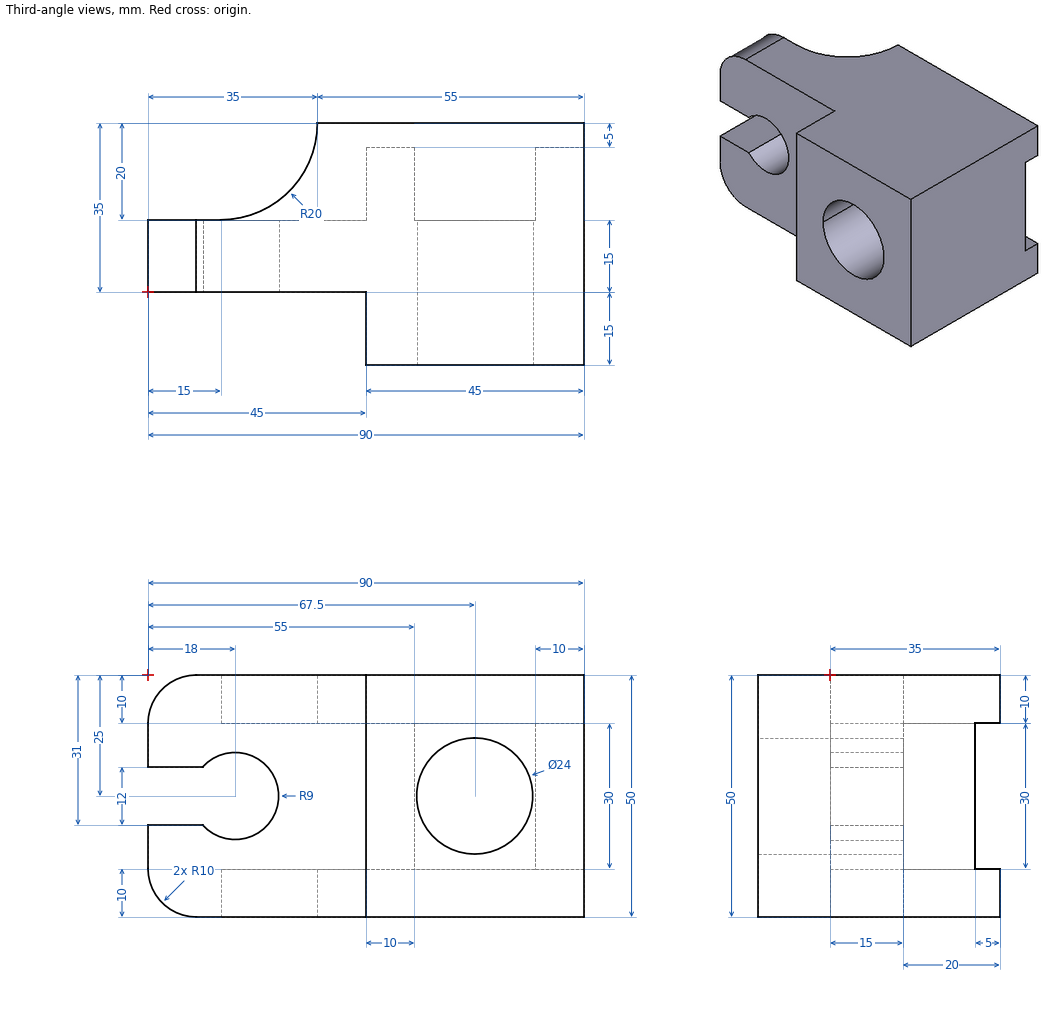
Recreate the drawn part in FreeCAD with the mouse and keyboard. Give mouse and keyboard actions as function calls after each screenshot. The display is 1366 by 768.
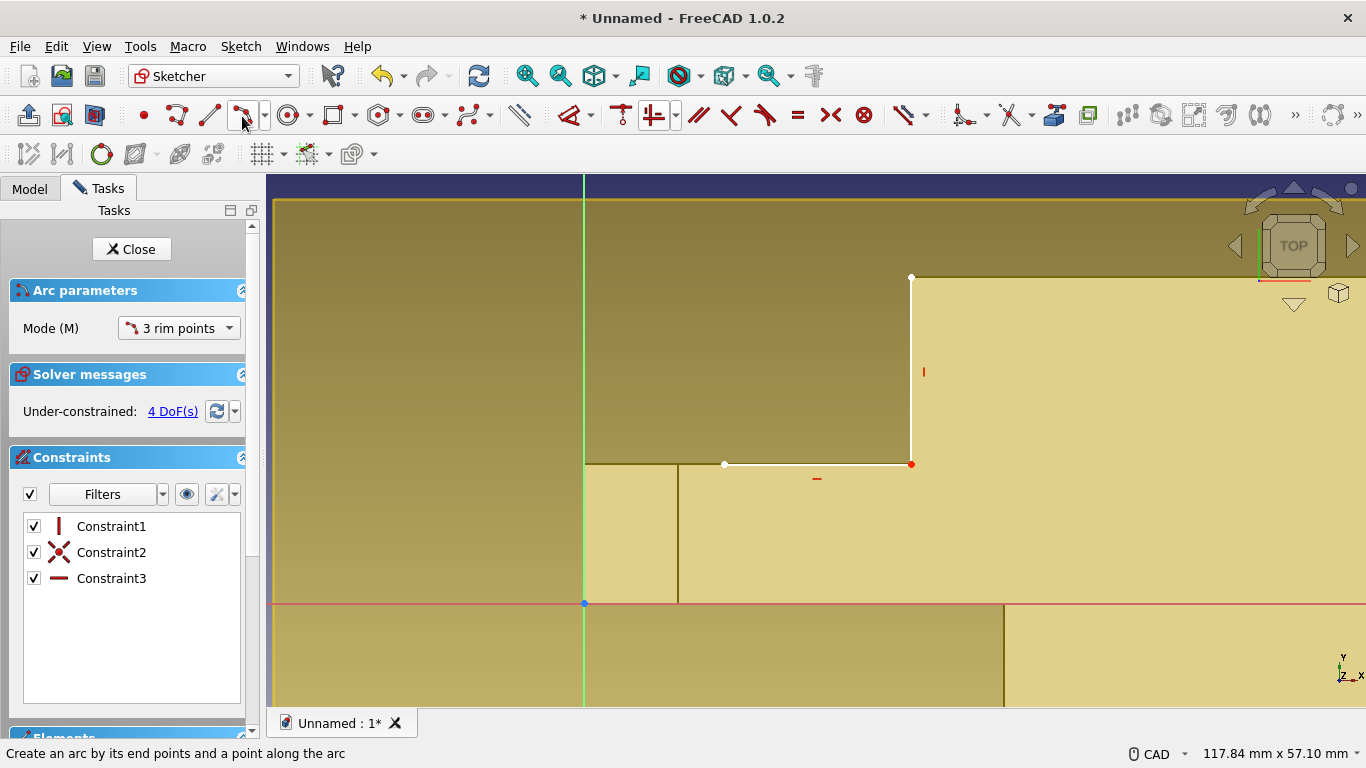
click(724, 465)
click(911, 278)
click(856, 409)
key(Escape)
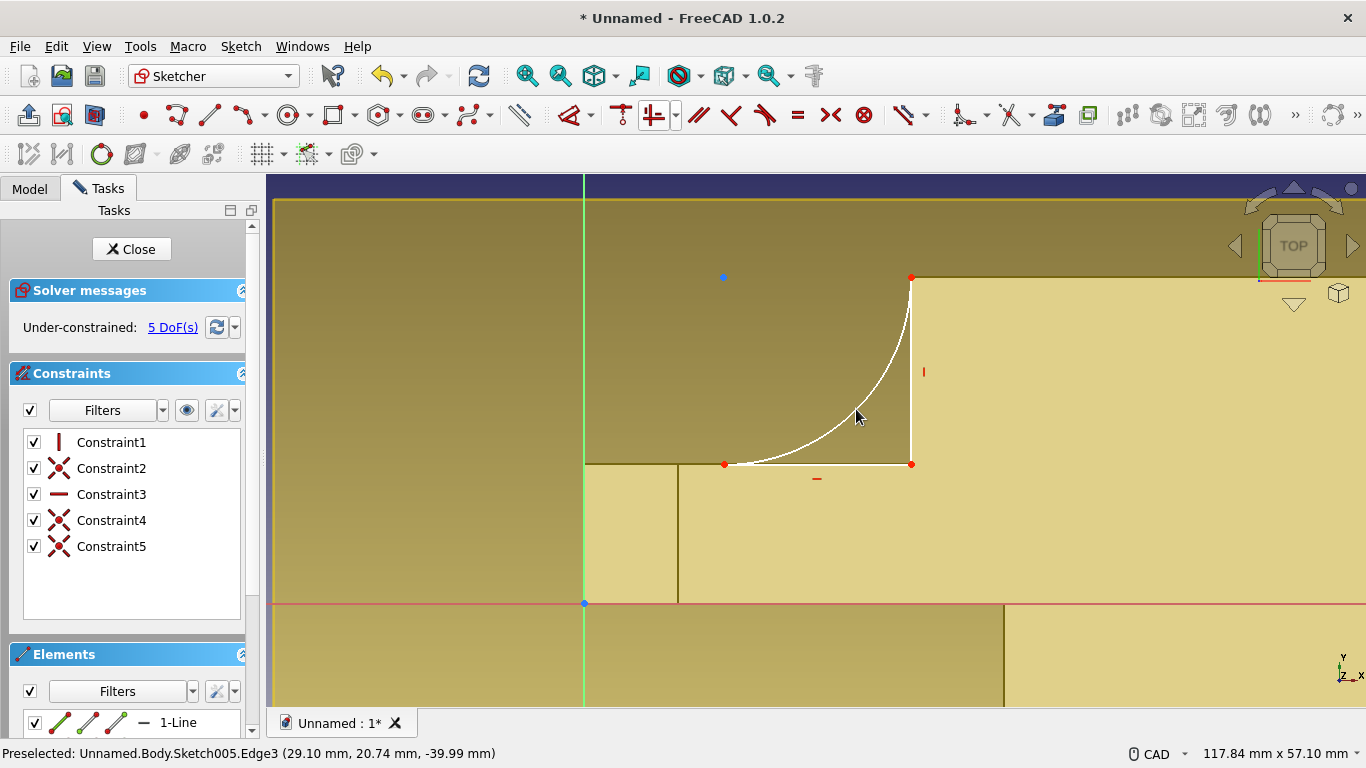
click(911, 409)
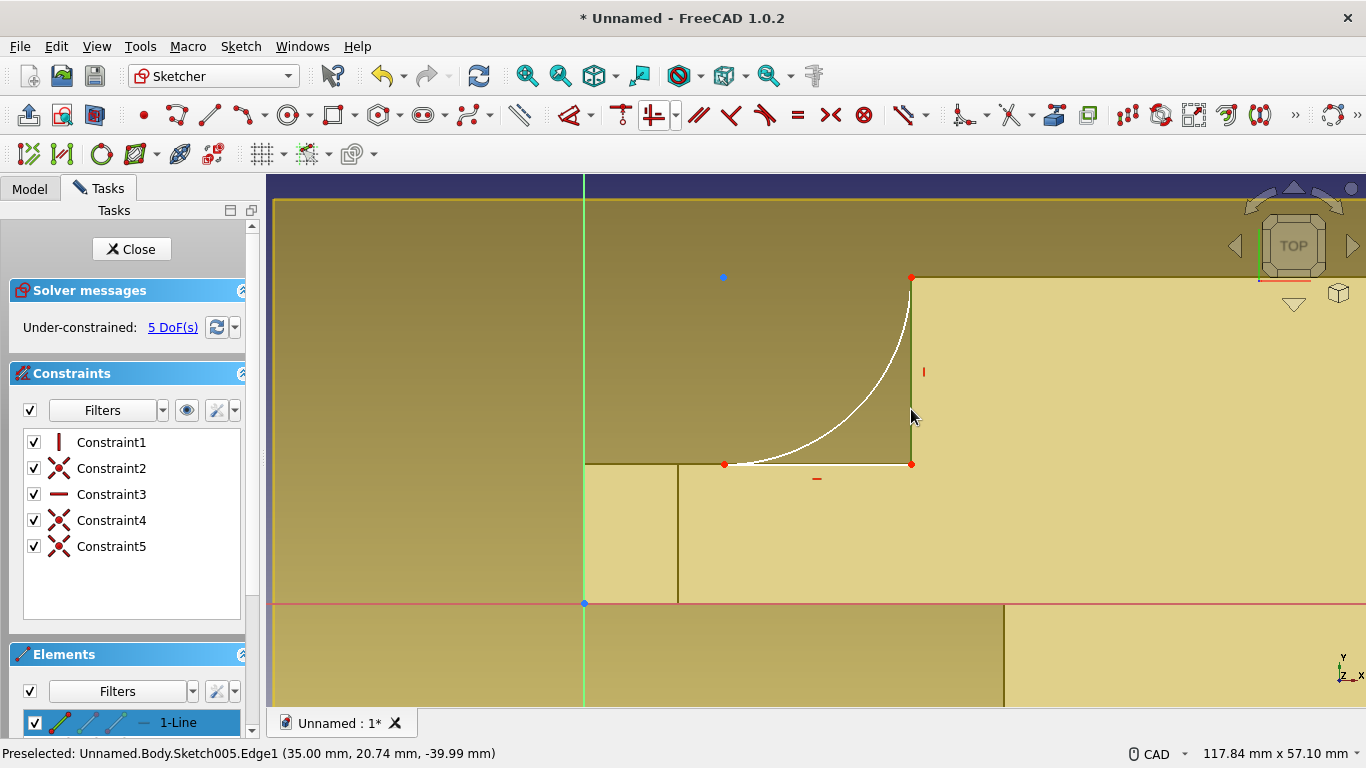
click(809, 444)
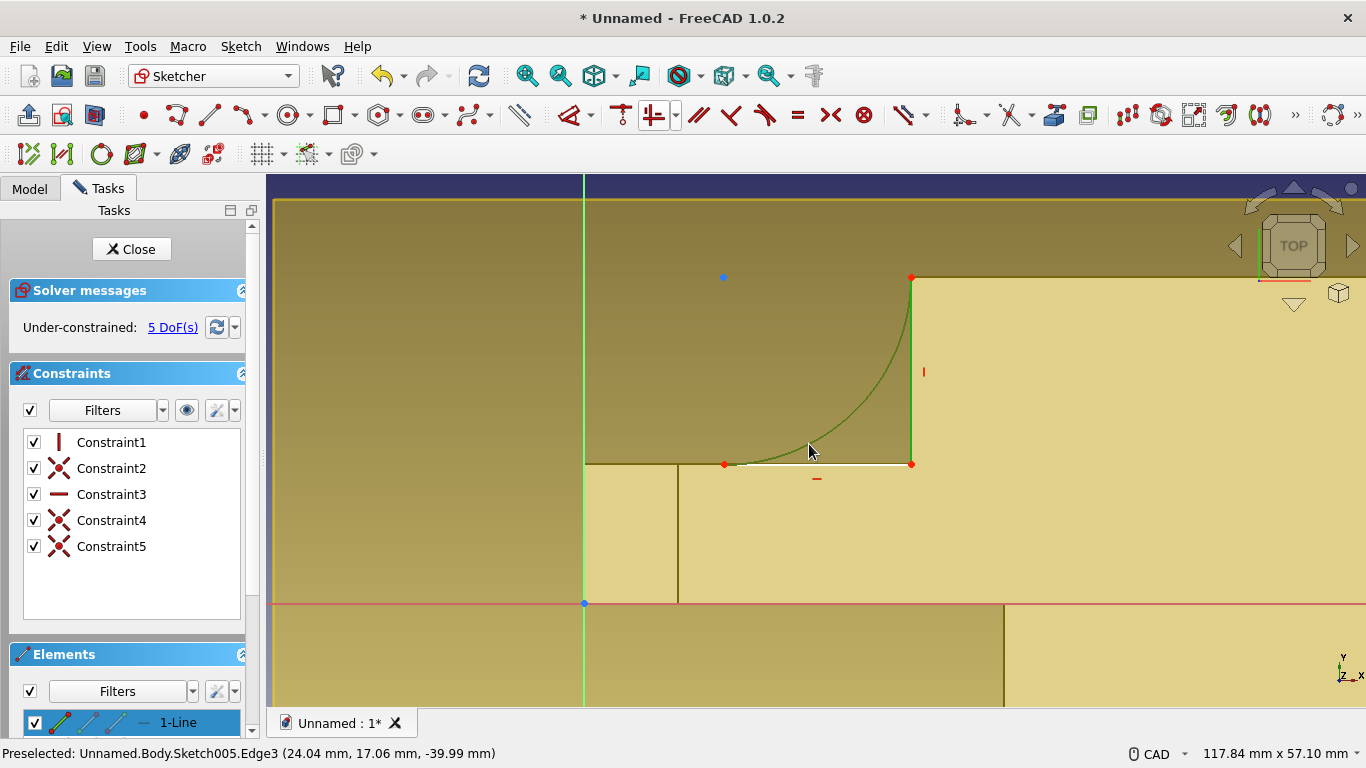
key(t)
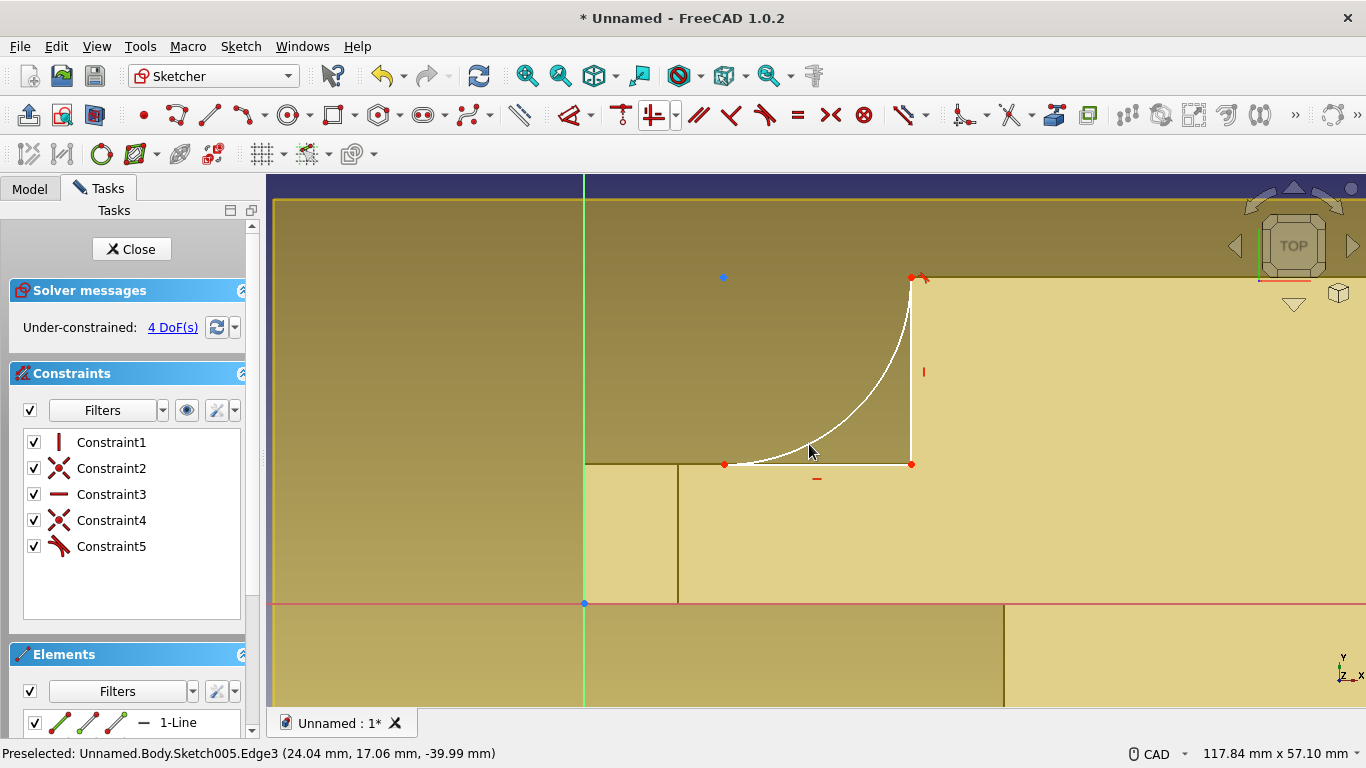
click(855, 465)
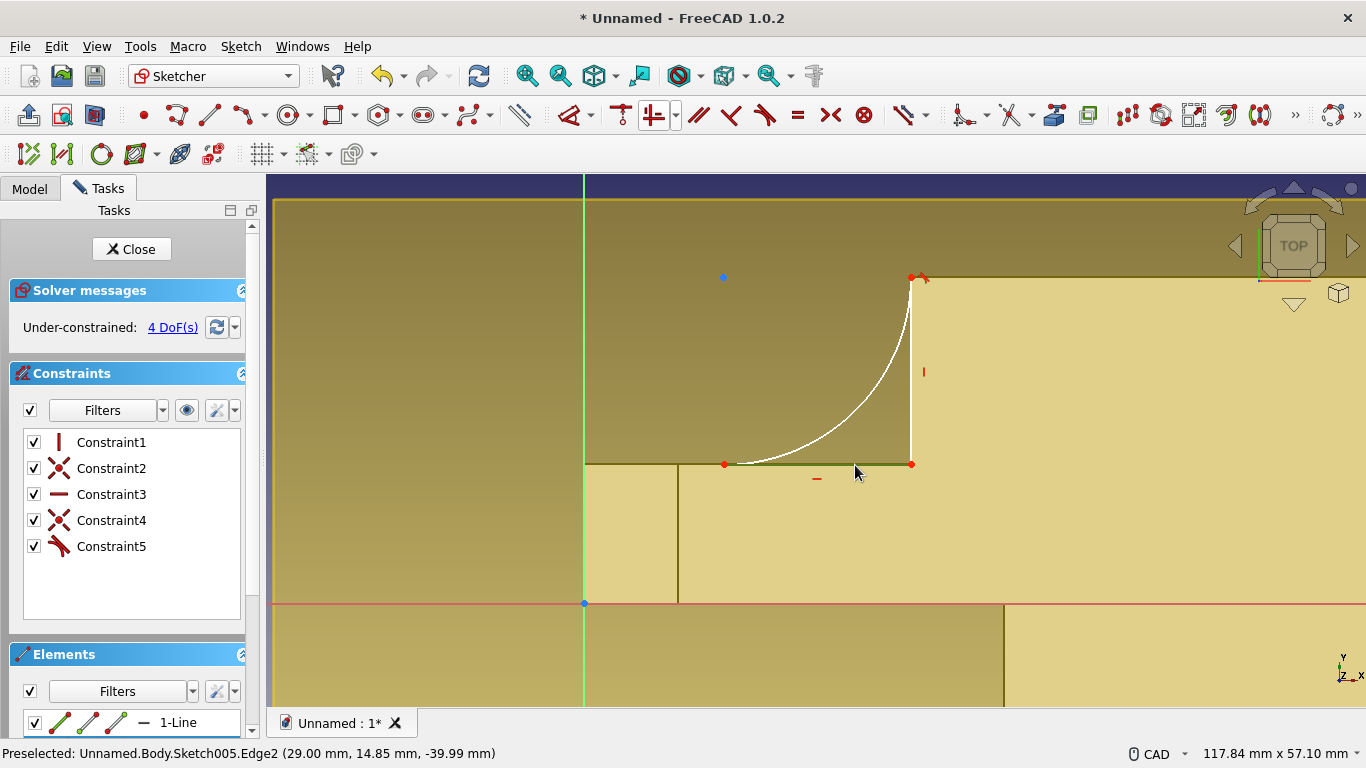
click(809, 444)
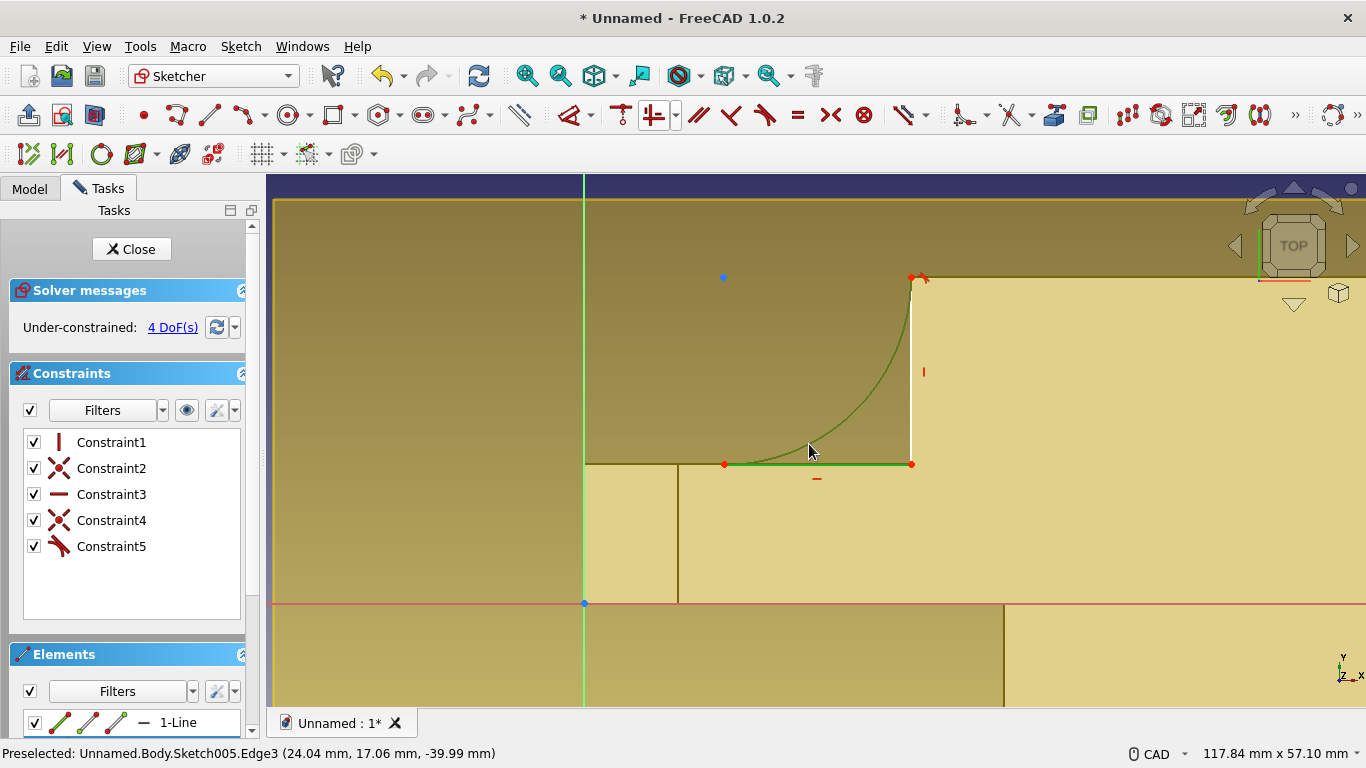
click(765, 116)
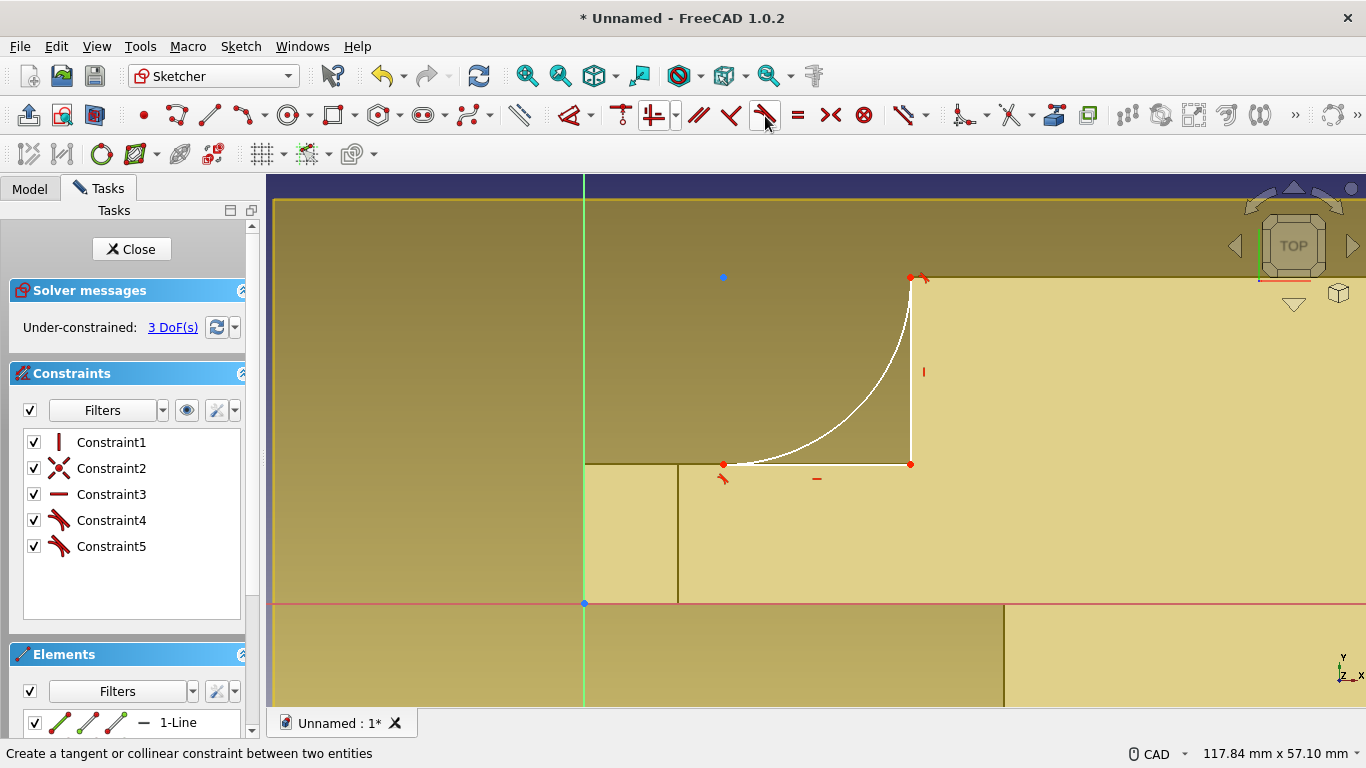
click(568, 116)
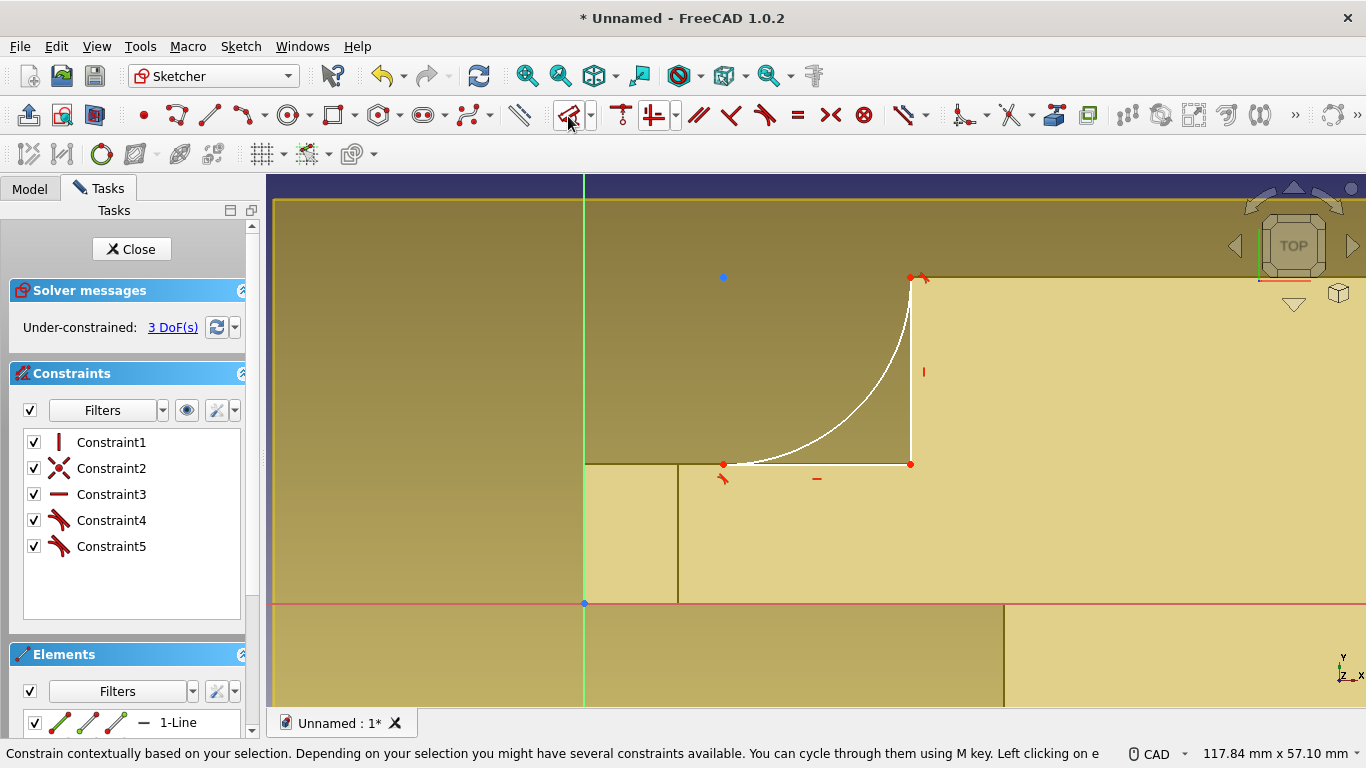
click(808, 445)
click(716, 497)